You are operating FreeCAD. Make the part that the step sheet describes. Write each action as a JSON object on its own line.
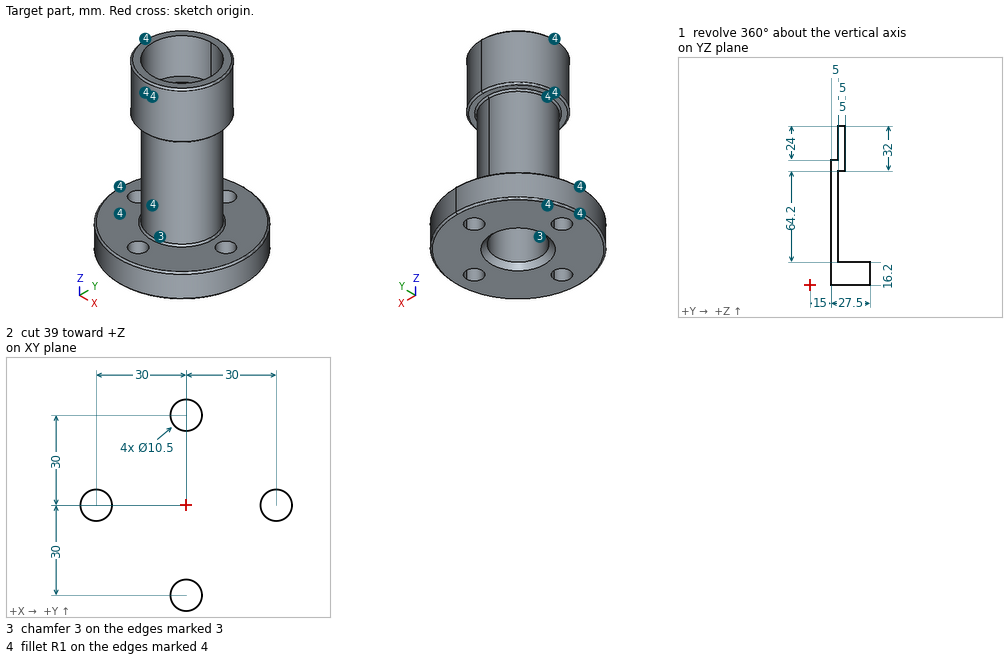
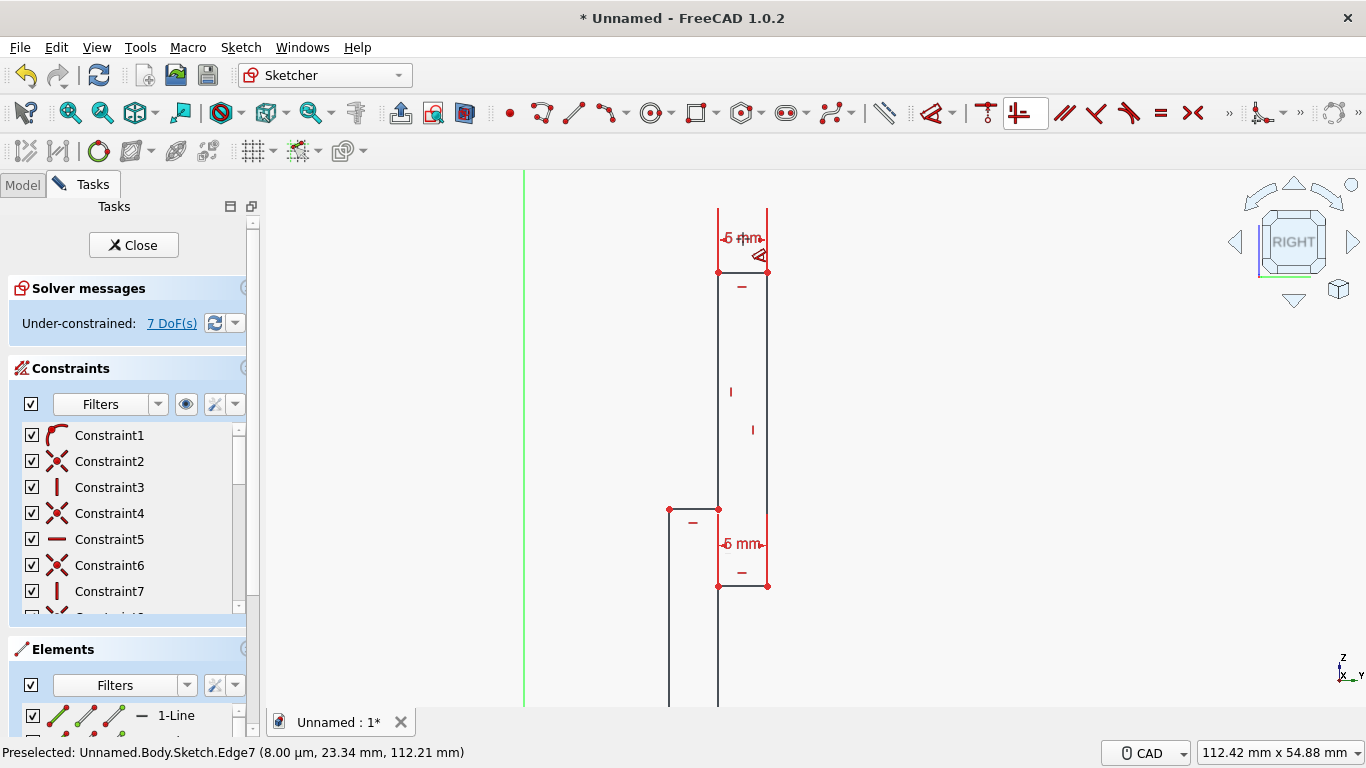
{"action": "left_click", "coordinate": [703, 509]}
{"action": "left_click", "coordinate": [694, 475]}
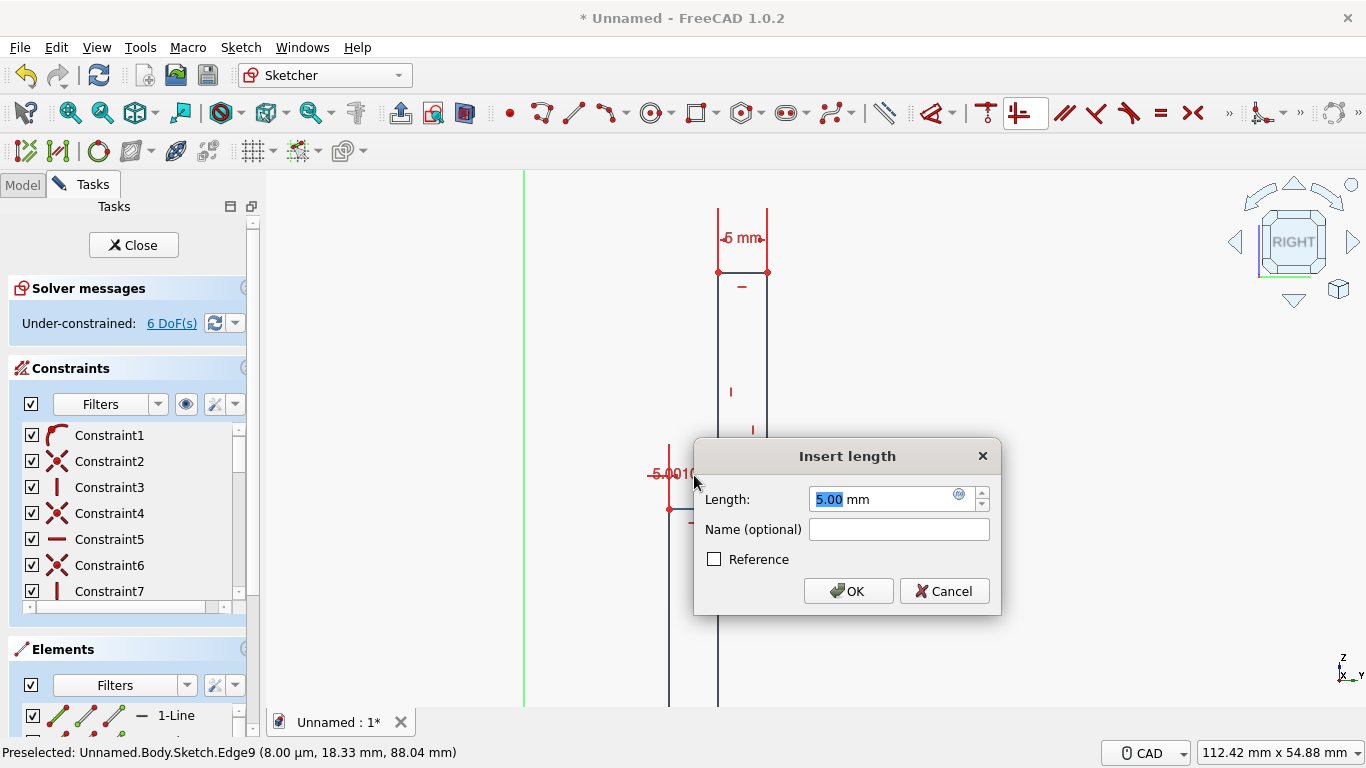
{"action": "type", "text": "5"}
{"action": "key", "text": "Return"}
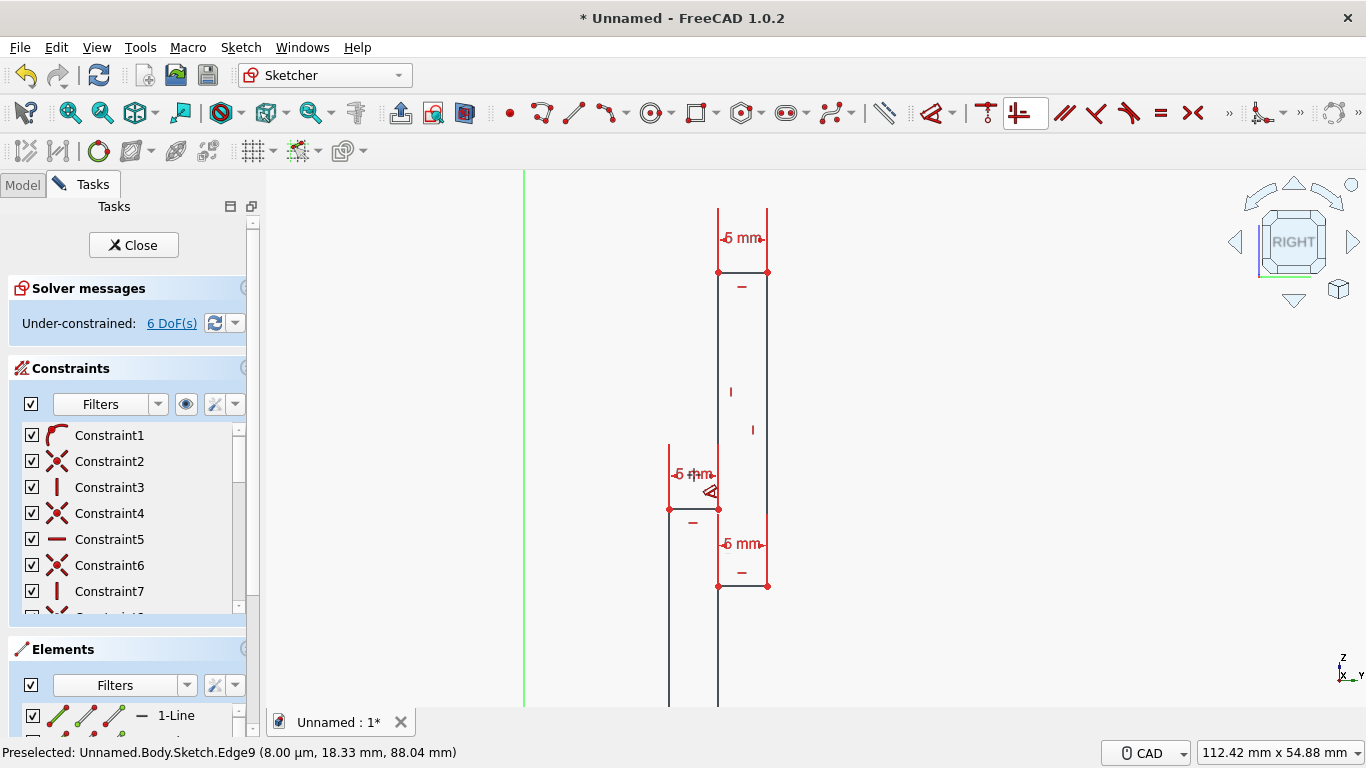
{"action": "scroll", "coordinate": [754, 274], "scroll_direction": "down", "scroll_amount": 6}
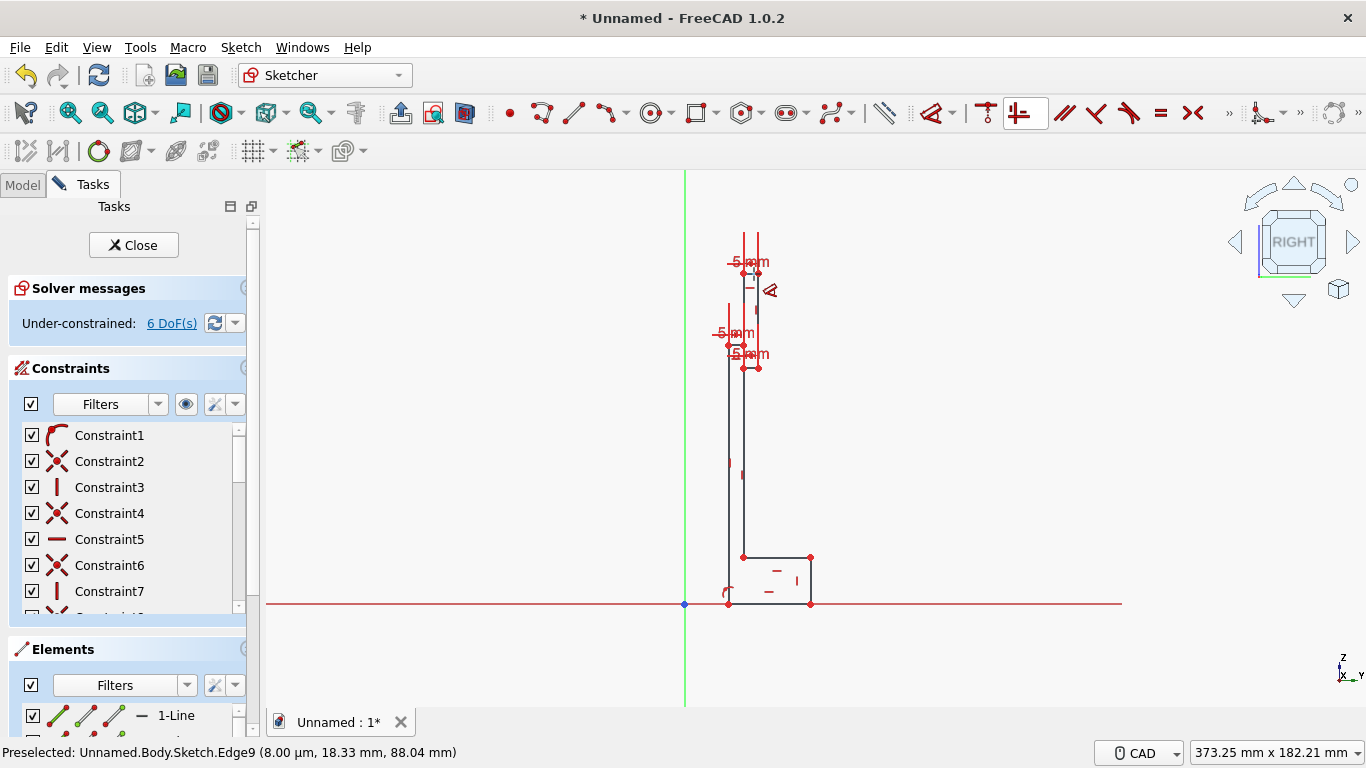
{"action": "left_click", "coordinate": [758, 340]}
{"action": "left_click", "coordinate": [792, 299]}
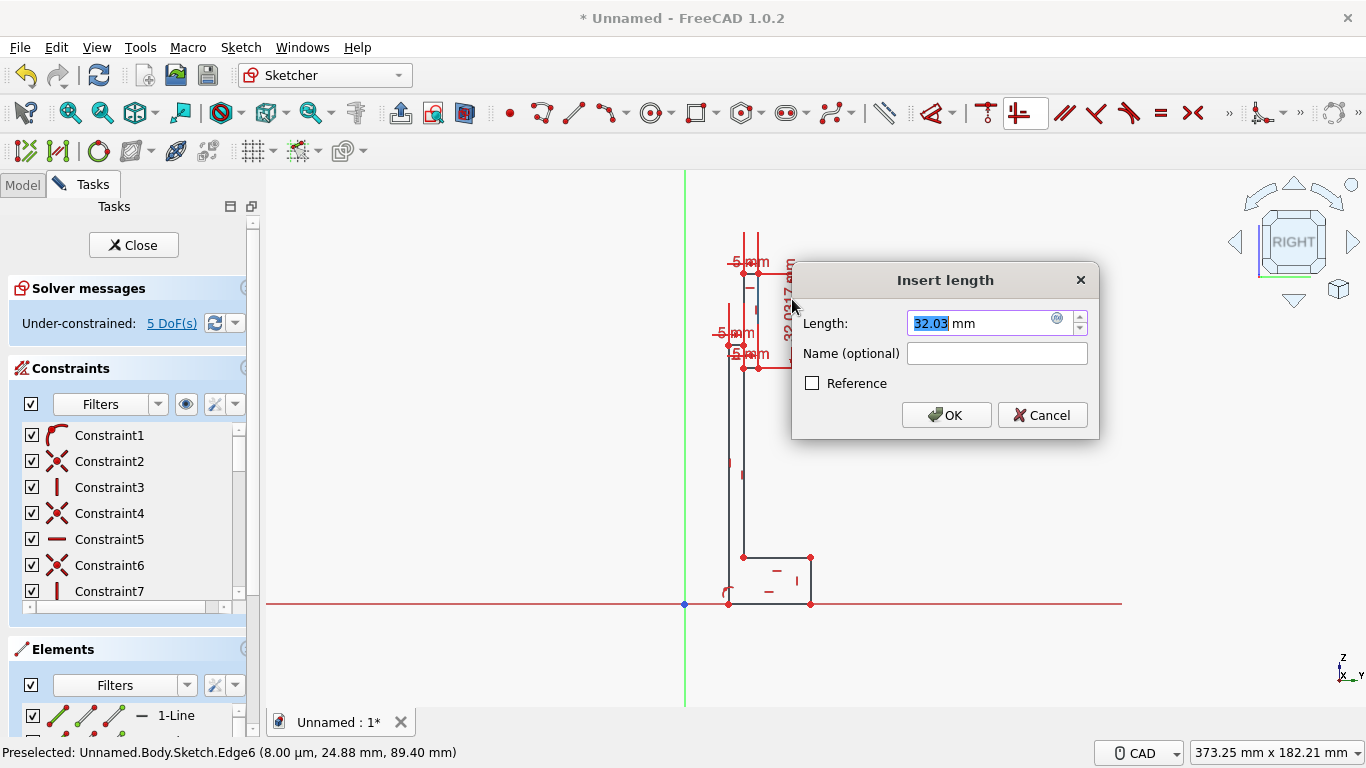
{"action": "type", "text": "32"}
{"action": "key", "text": "Return"}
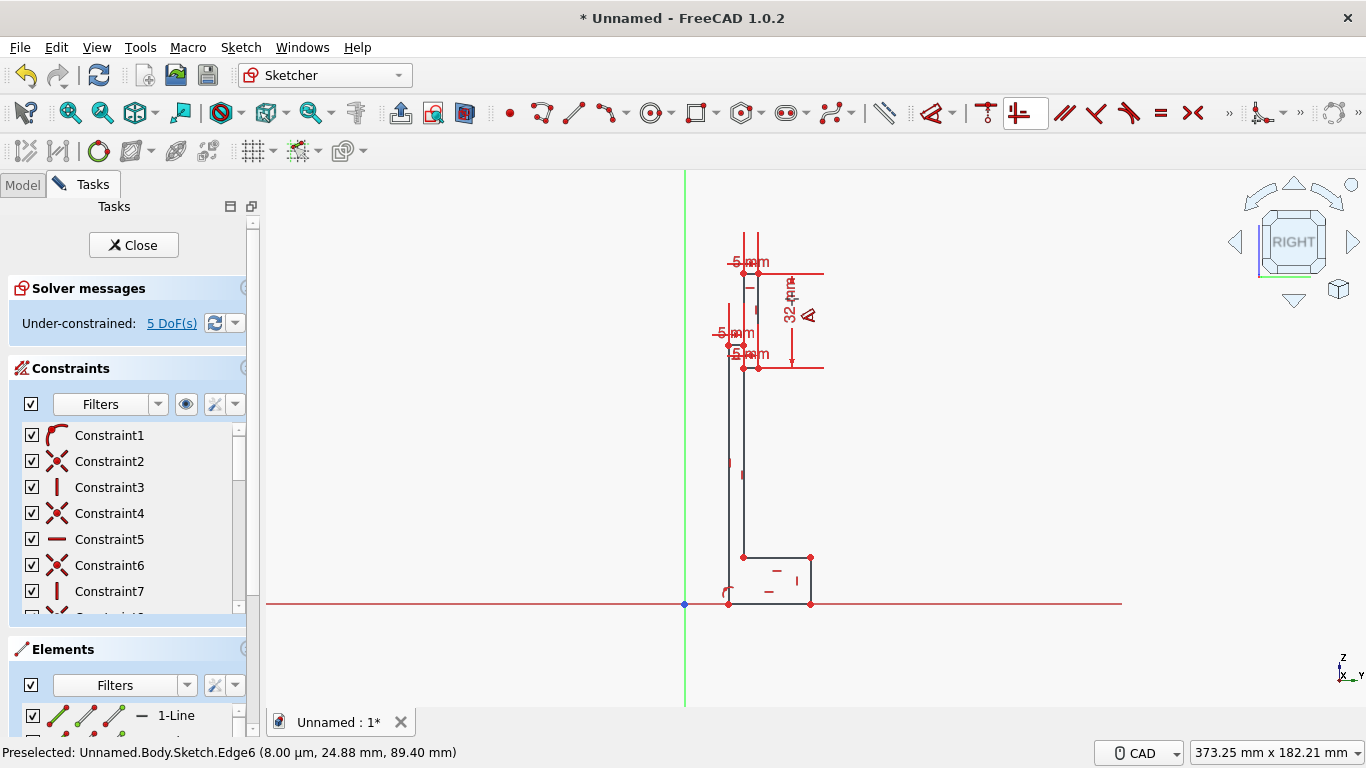
{"action": "left_click", "coordinate": [744, 295]}
{"action": "left_click", "coordinate": [710, 309]}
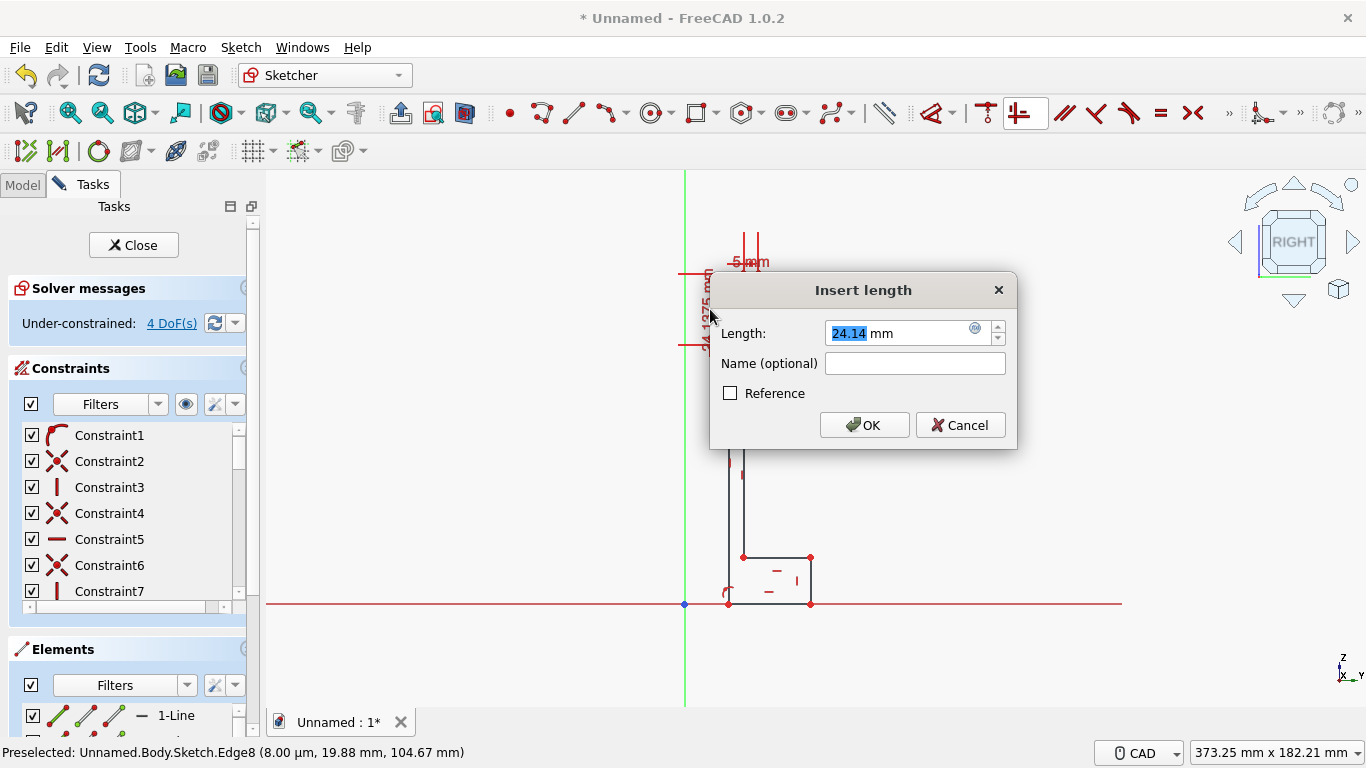
{"action": "type", "text": "24"}
{"action": "key", "text": "Return"}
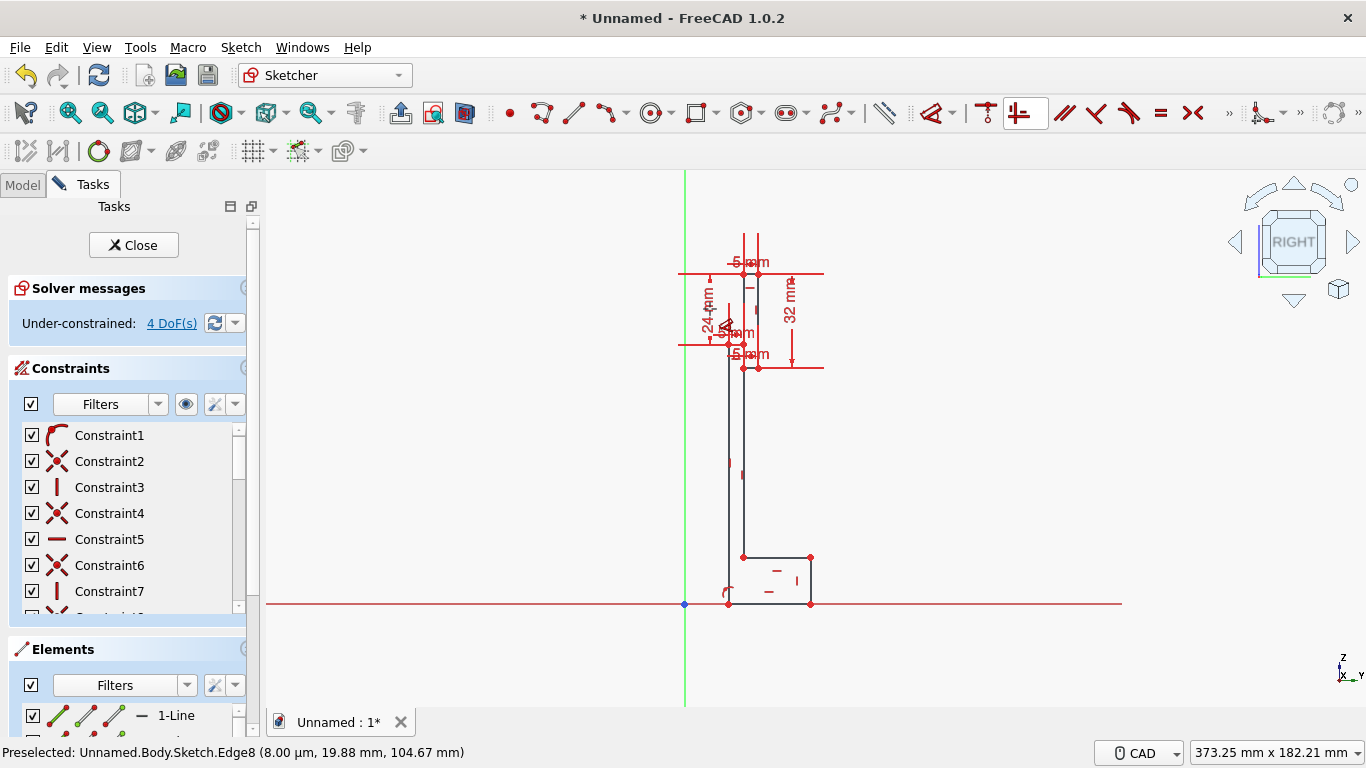
{"action": "left_click", "coordinate": [729, 604]}
{"action": "left_click", "coordinate": [707, 638]}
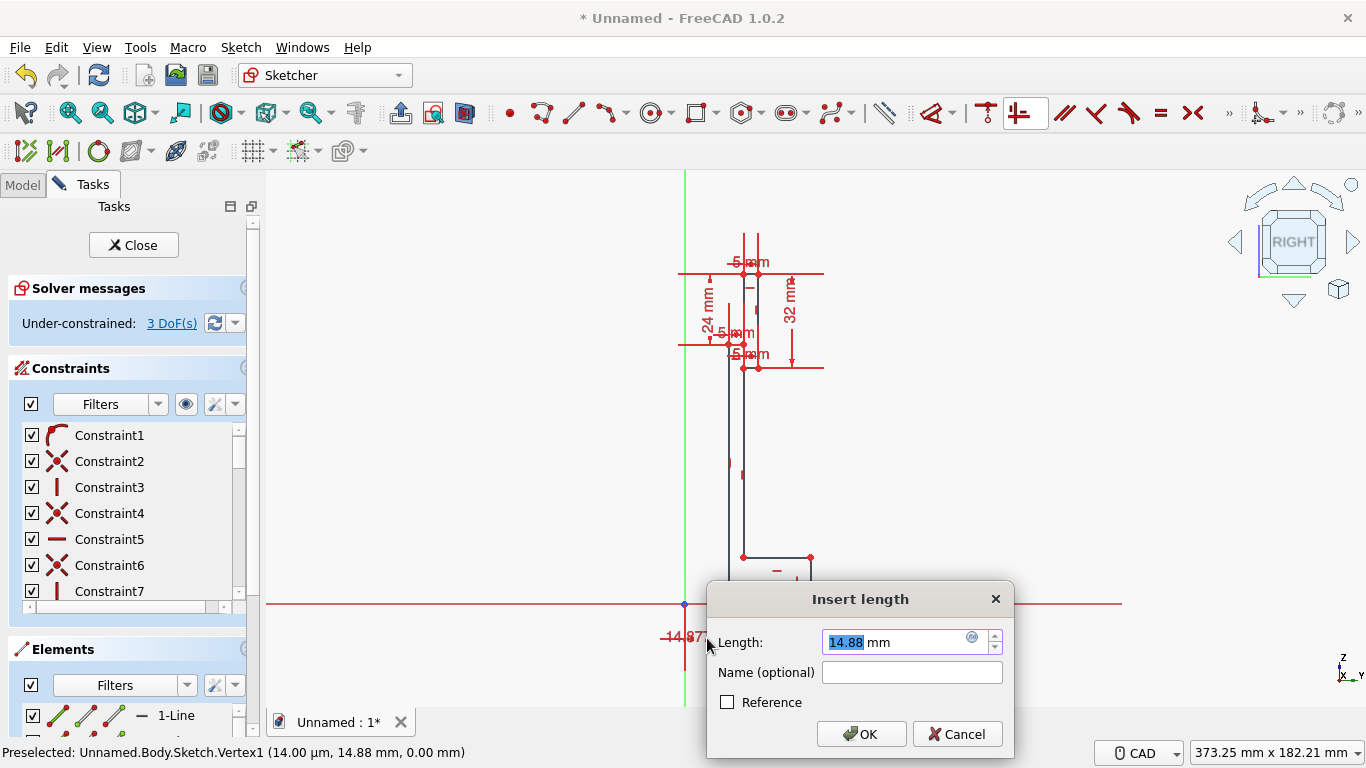
{"action": "type", "text": "15"}
{"action": "key", "text": "Return"}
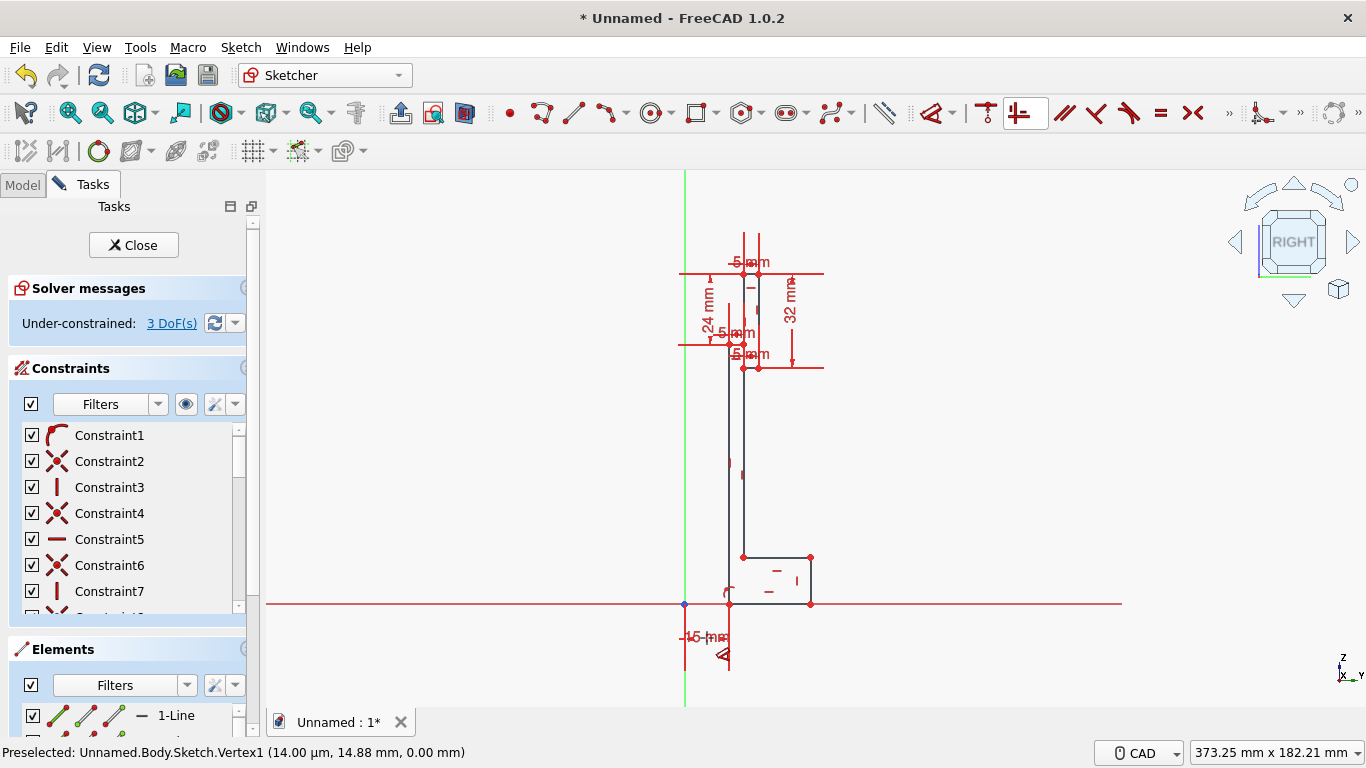
{"action": "left_click", "coordinate": [754, 604]}
{"action": "left_click", "coordinate": [789, 638]}